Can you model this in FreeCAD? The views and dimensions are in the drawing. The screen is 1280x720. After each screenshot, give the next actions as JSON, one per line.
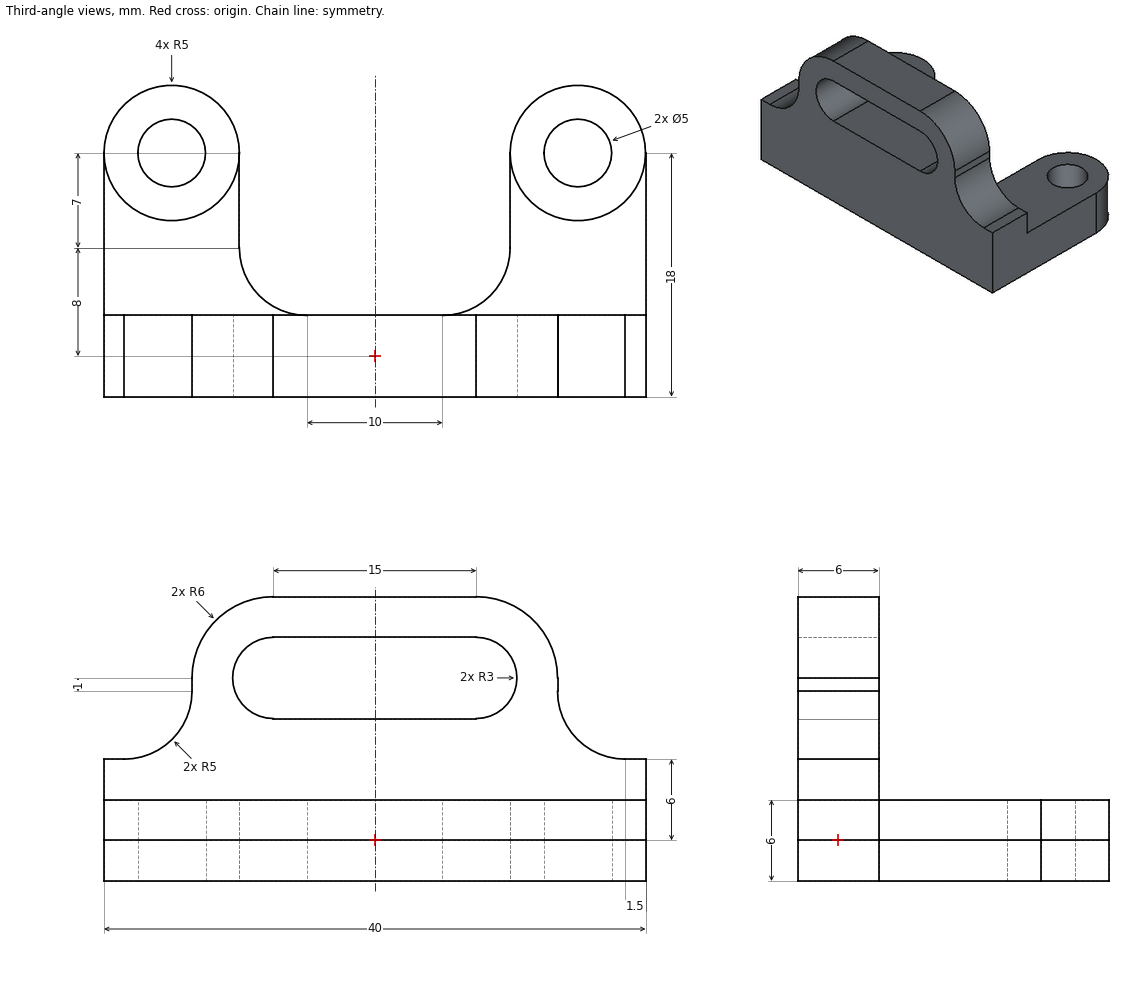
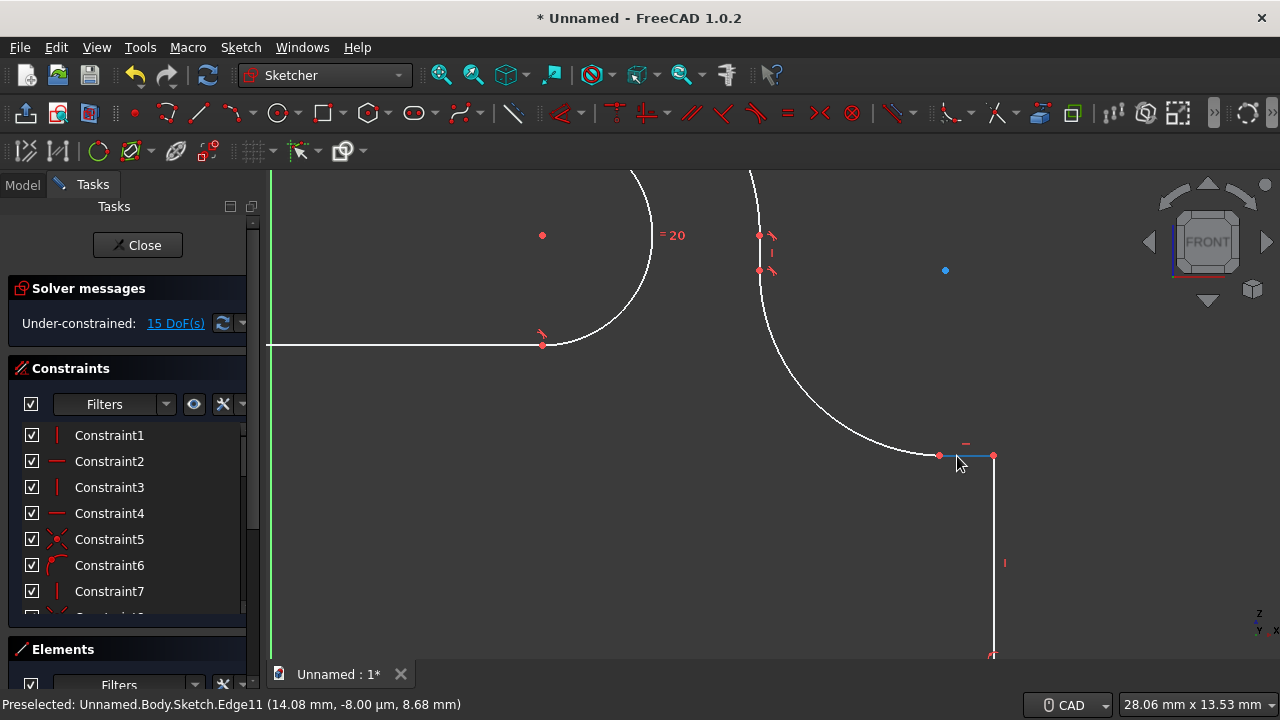
{"action": "left_click", "coordinate": [956, 456]}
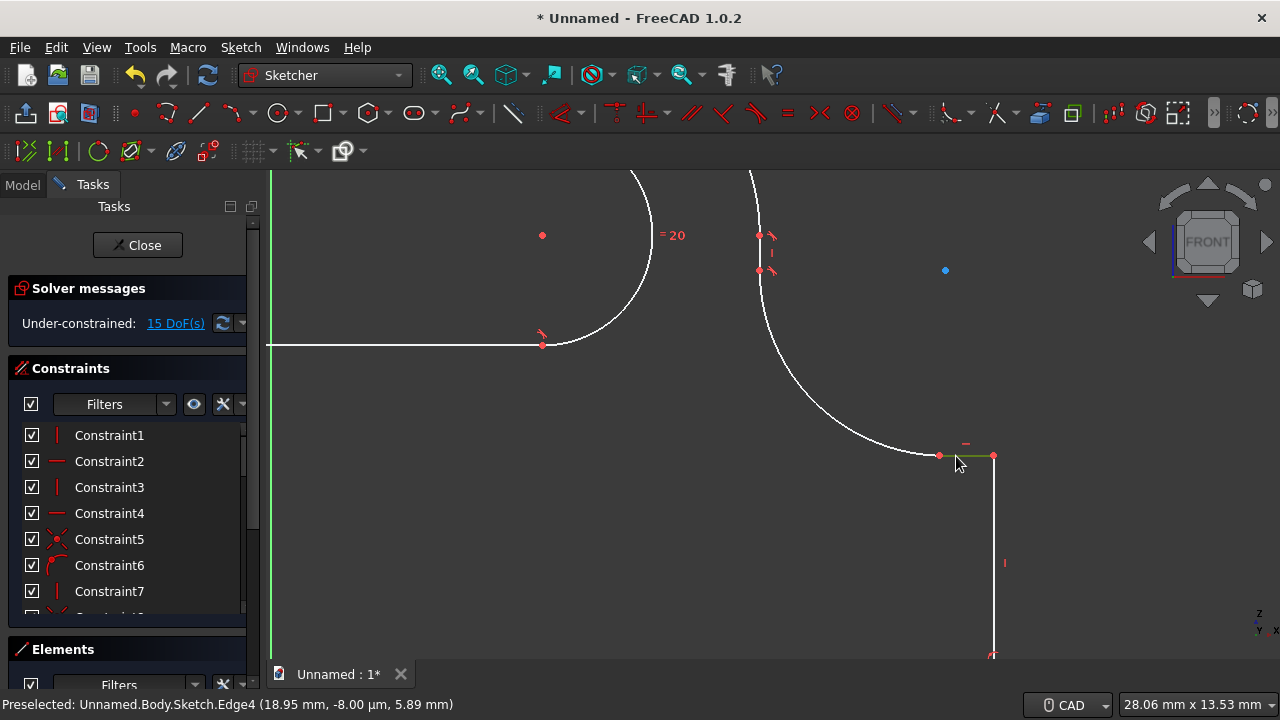
{"action": "left_click", "coordinate": [779, 353]}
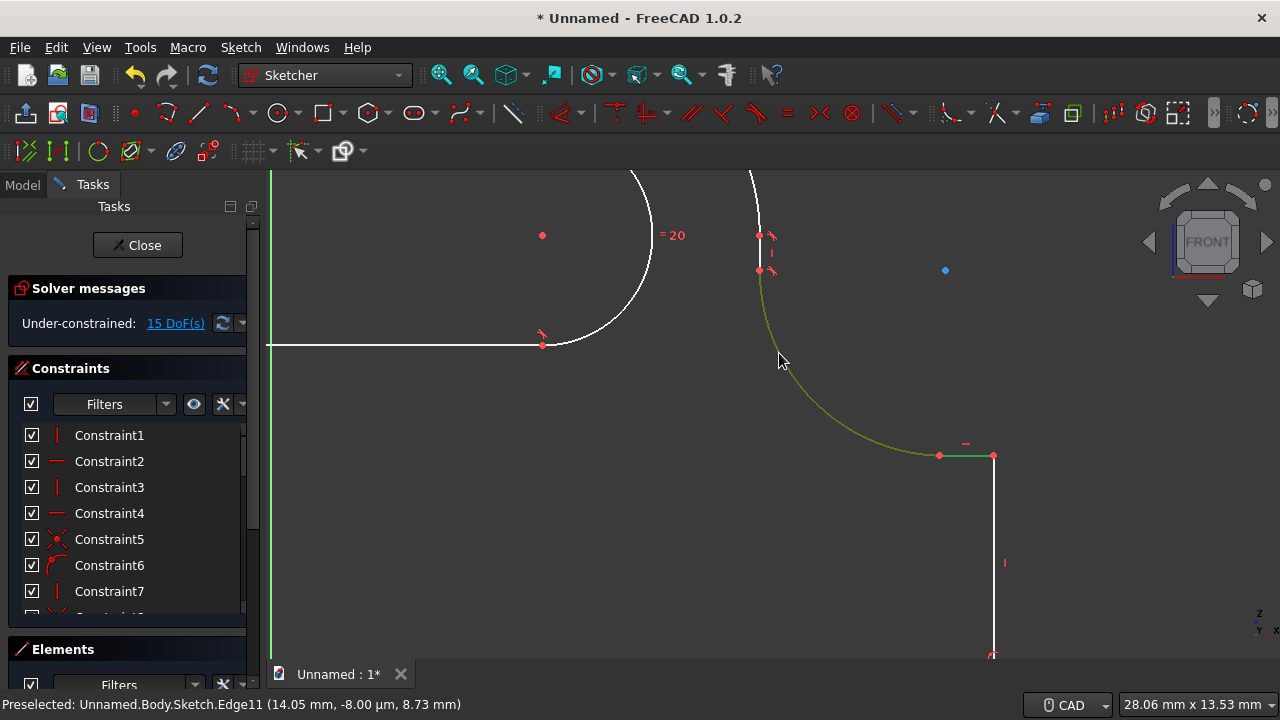
{"action": "left_click", "coordinate": [756, 114]}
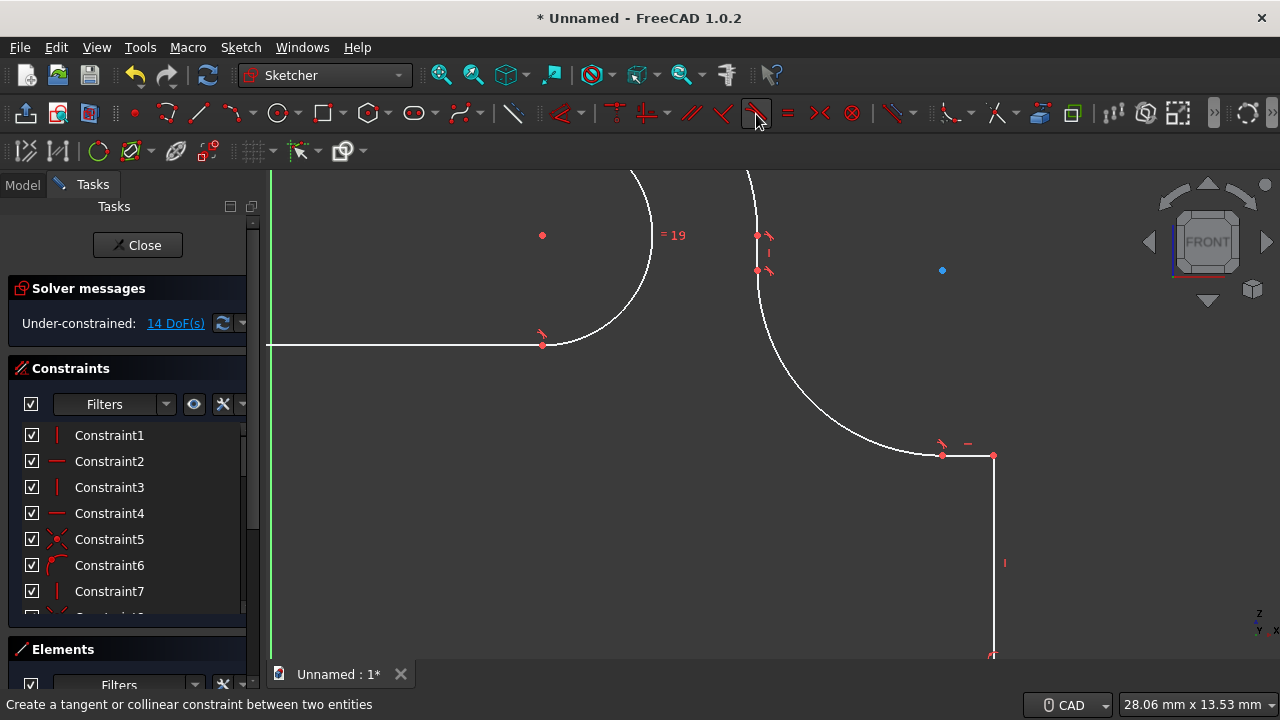
{"action": "scroll", "coordinate": [957, 456], "scroll_direction": "down", "scroll_amount": 5}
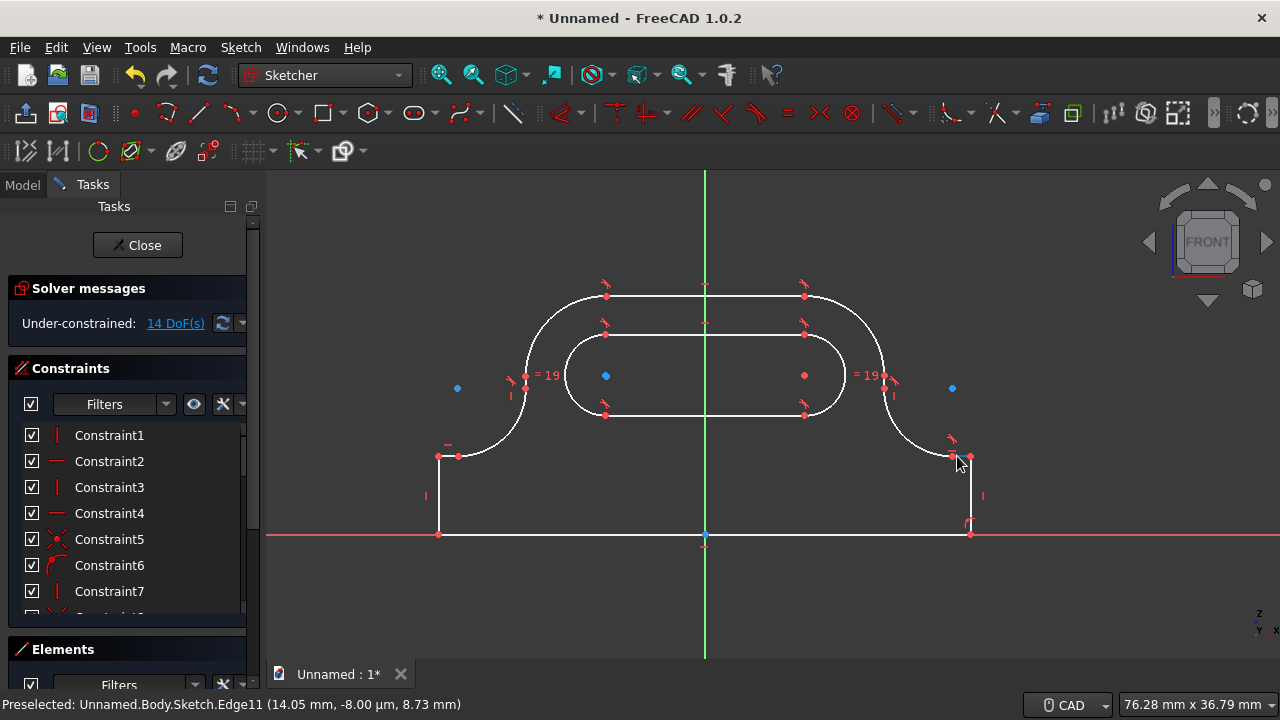
{"action": "scroll", "coordinate": [445, 456], "scroll_direction": "up", "scroll_amount": 5}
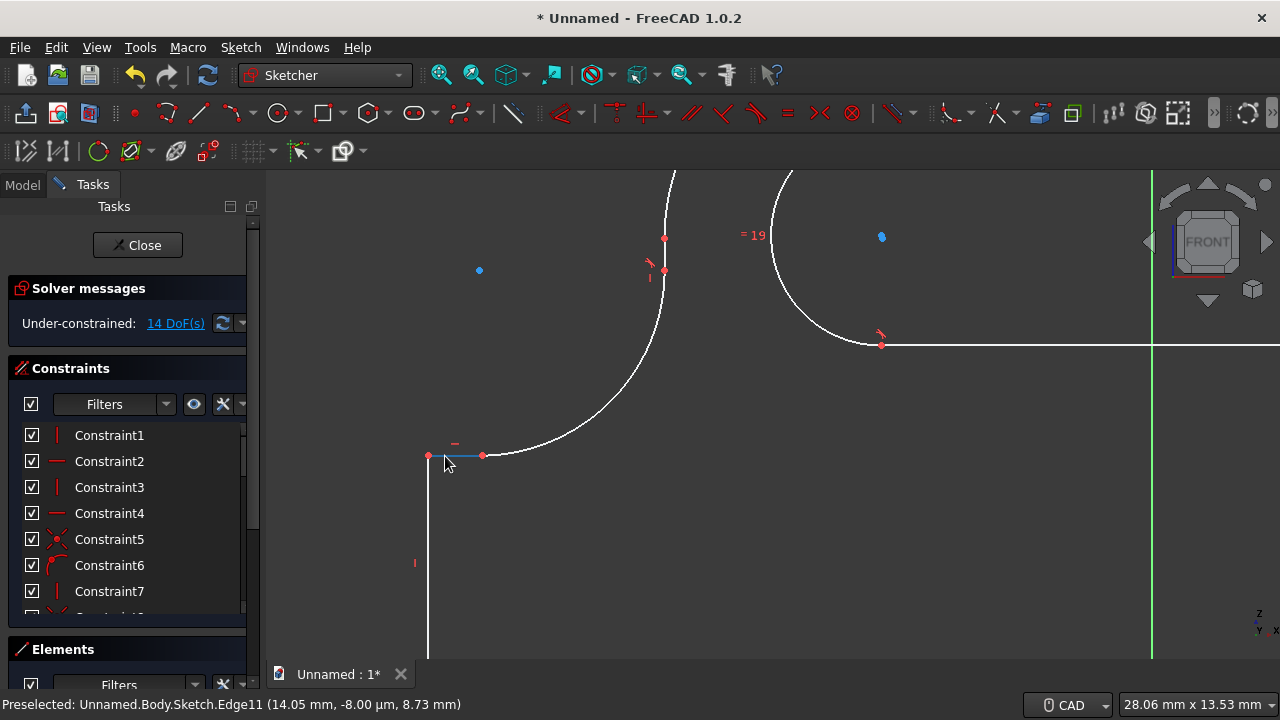
{"action": "left_click", "coordinate": [444, 456]}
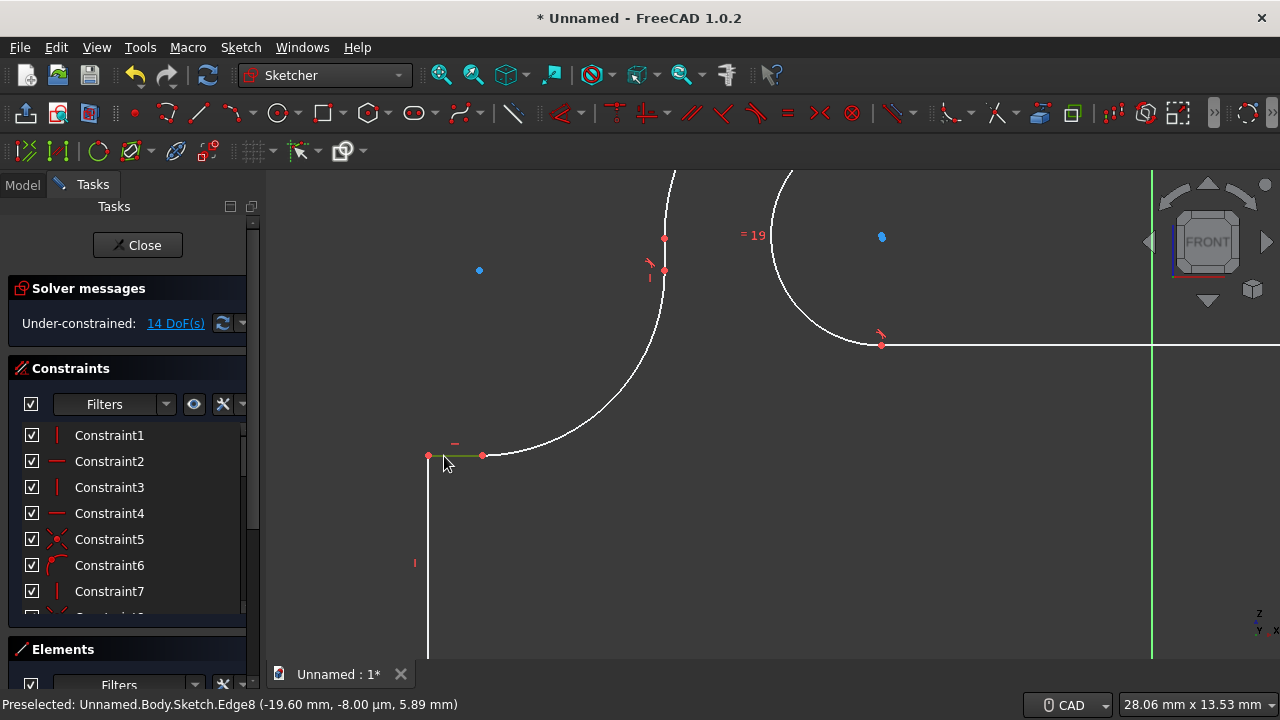
{"action": "left_click", "coordinate": [565, 435]}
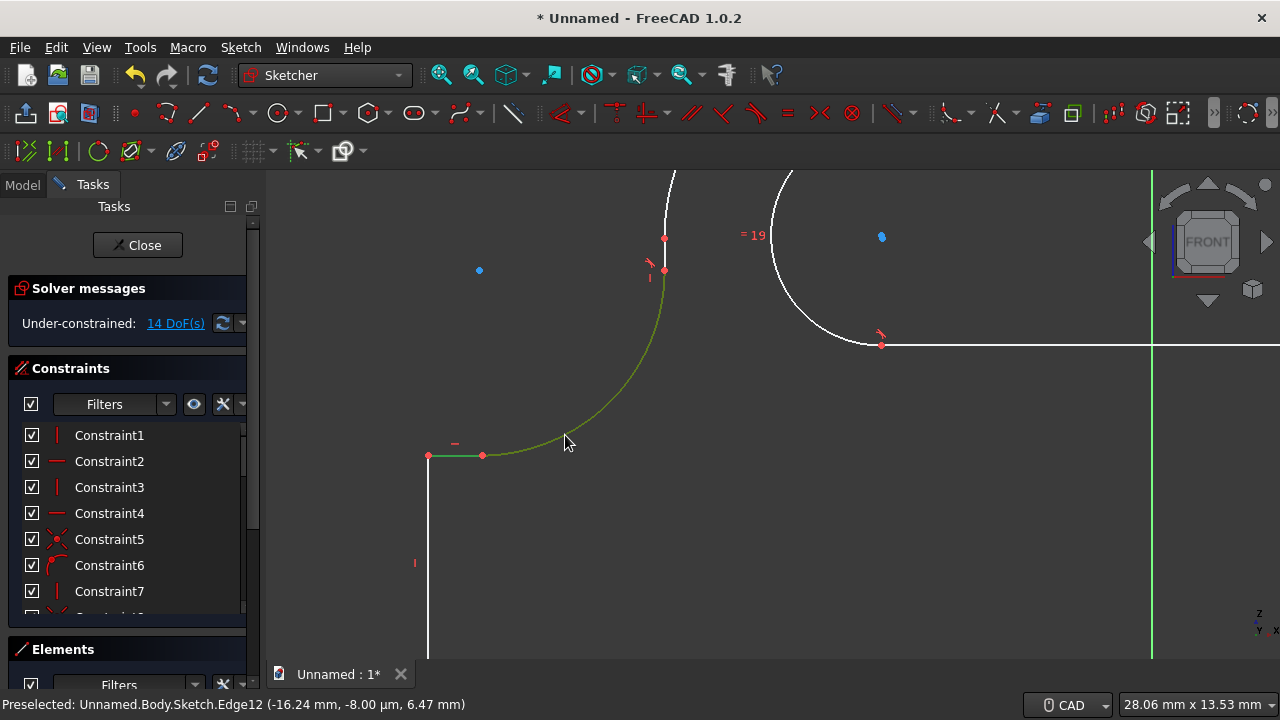
{"action": "left_click", "coordinate": [756, 114]}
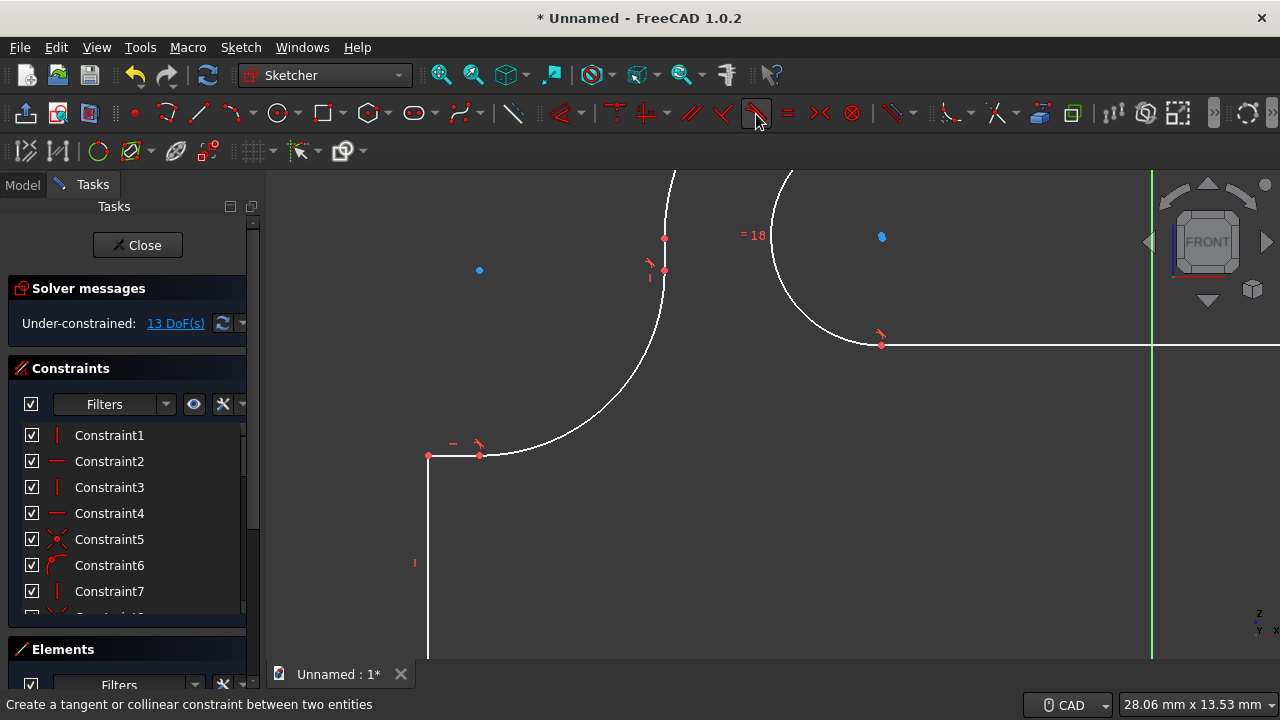
{"action": "scroll", "coordinate": [444, 456], "scroll_direction": "down", "scroll_amount": 5}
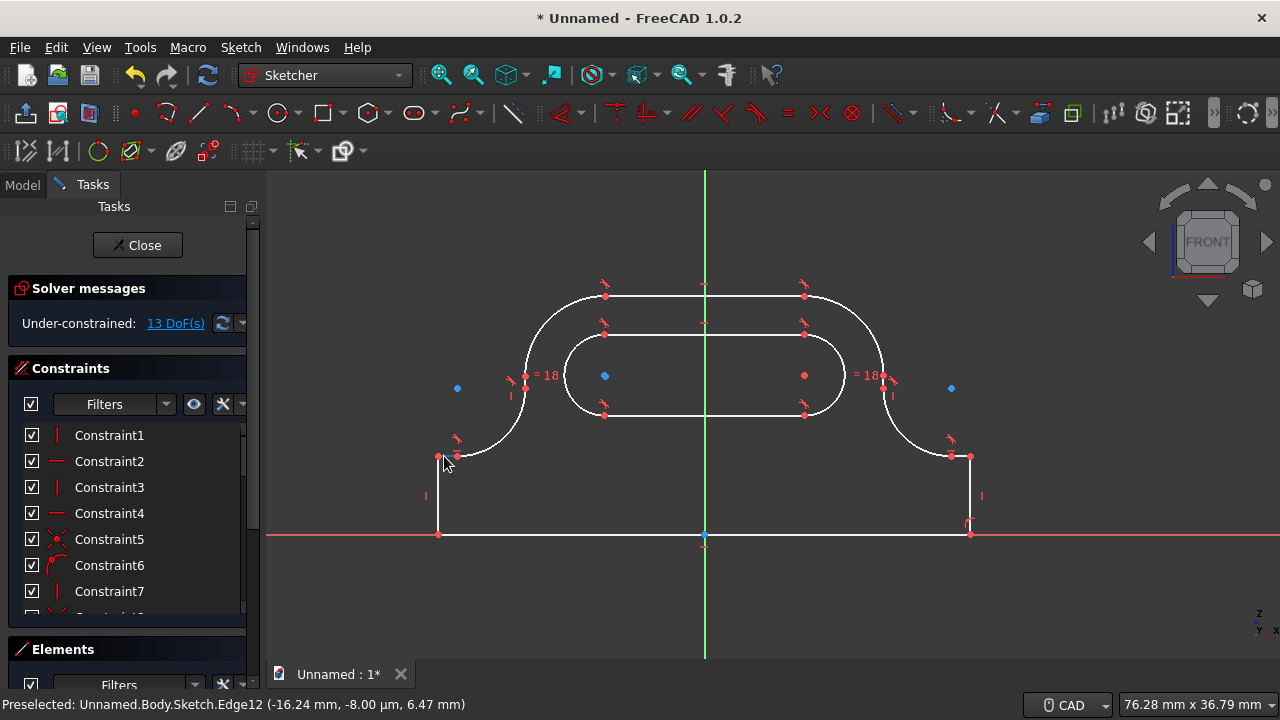
{"action": "left_click", "coordinate": [569, 305]}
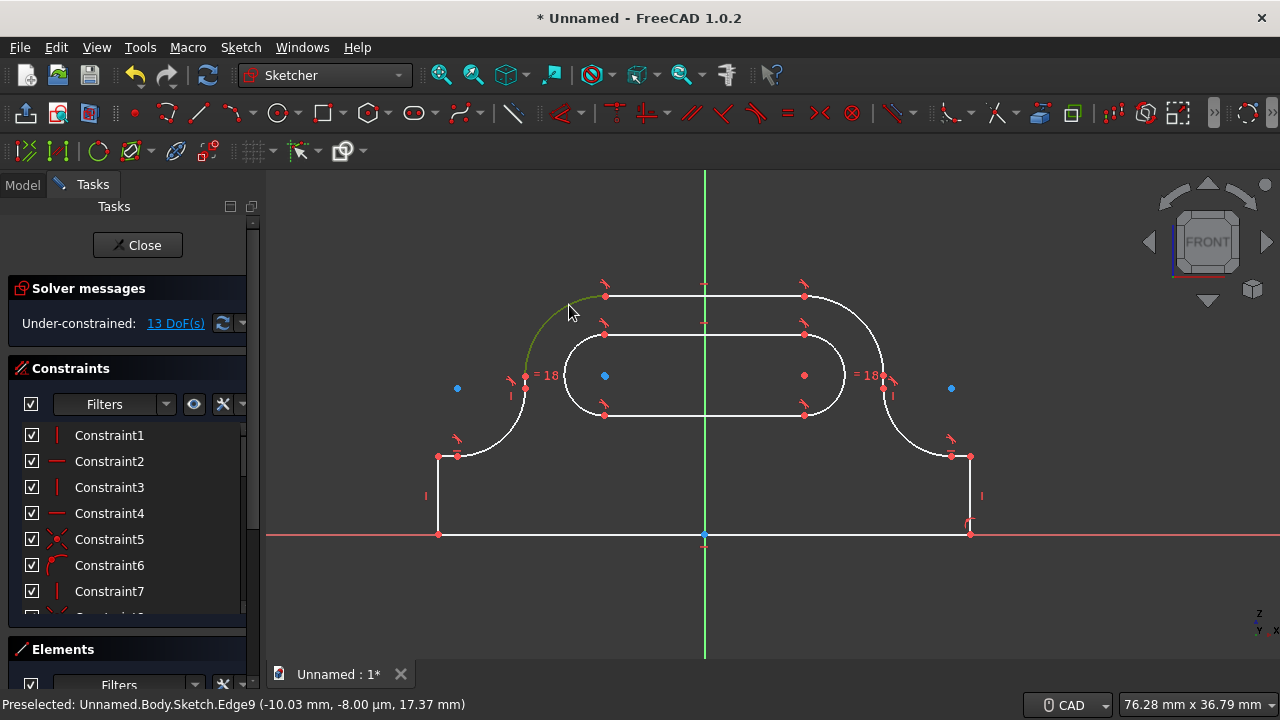
{"action": "left_click", "coordinate": [572, 351]}